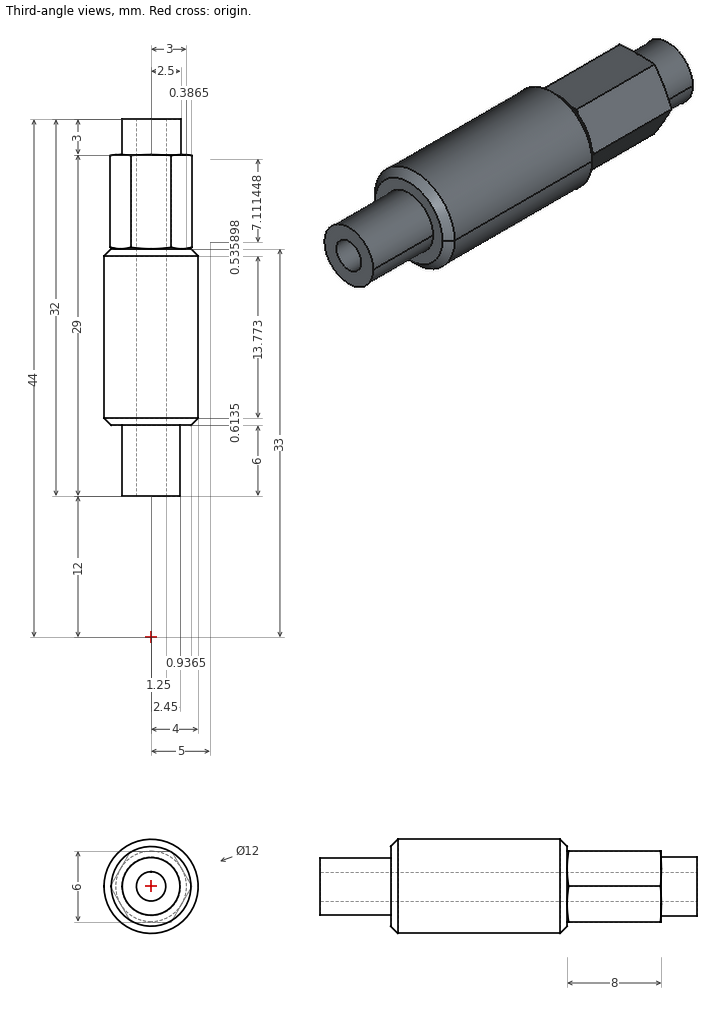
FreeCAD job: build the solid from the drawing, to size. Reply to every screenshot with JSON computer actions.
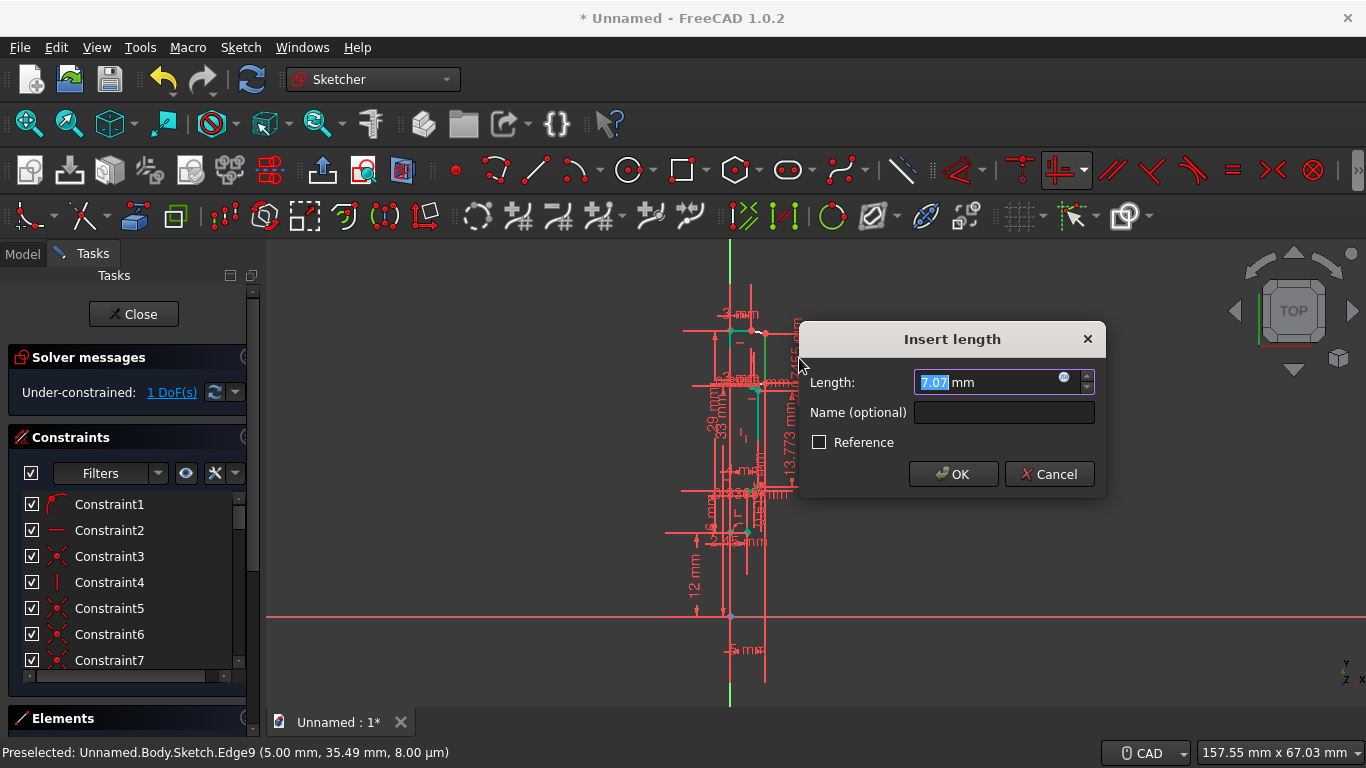
{"action": "type", "text": "7.111448"}
{"action": "key", "text": "Return"}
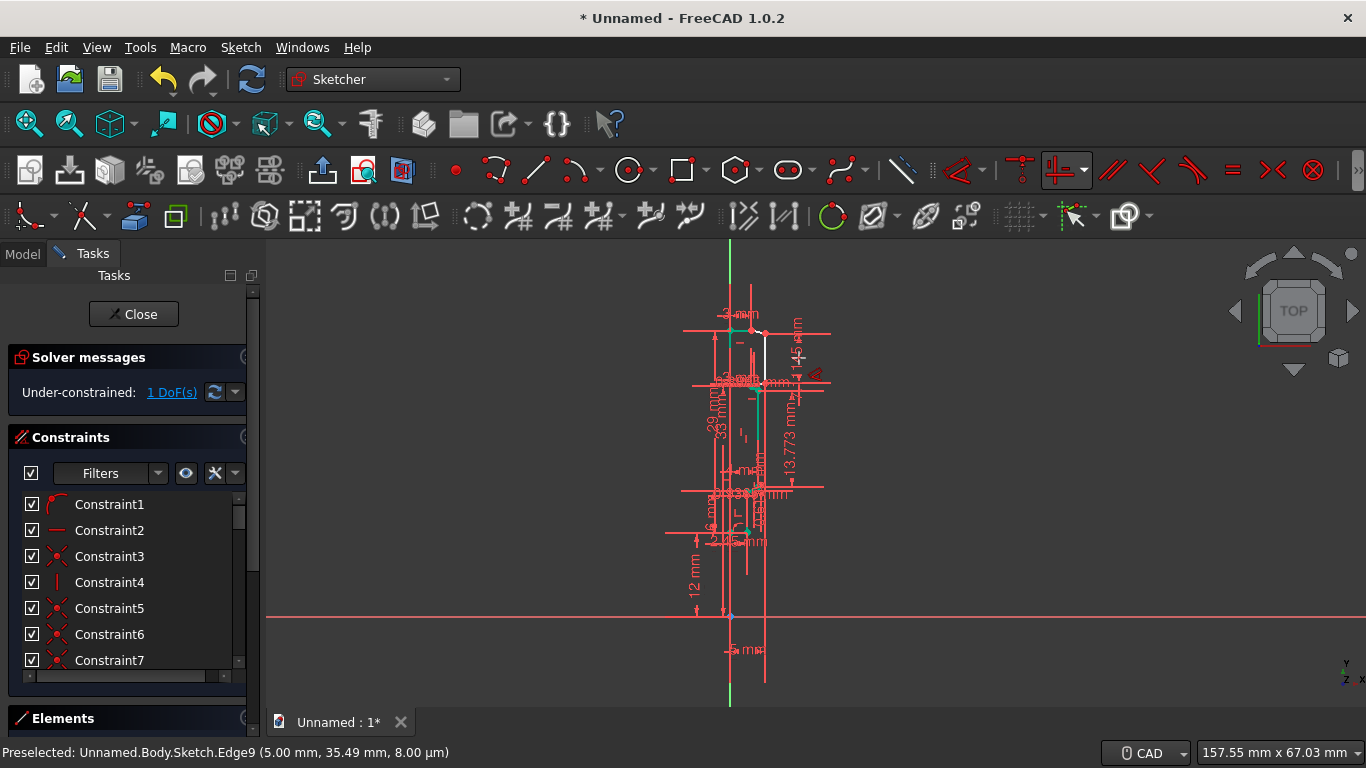
{"action": "scroll", "coordinate": [760, 384], "scroll_direction": "up", "scroll_amount": 12}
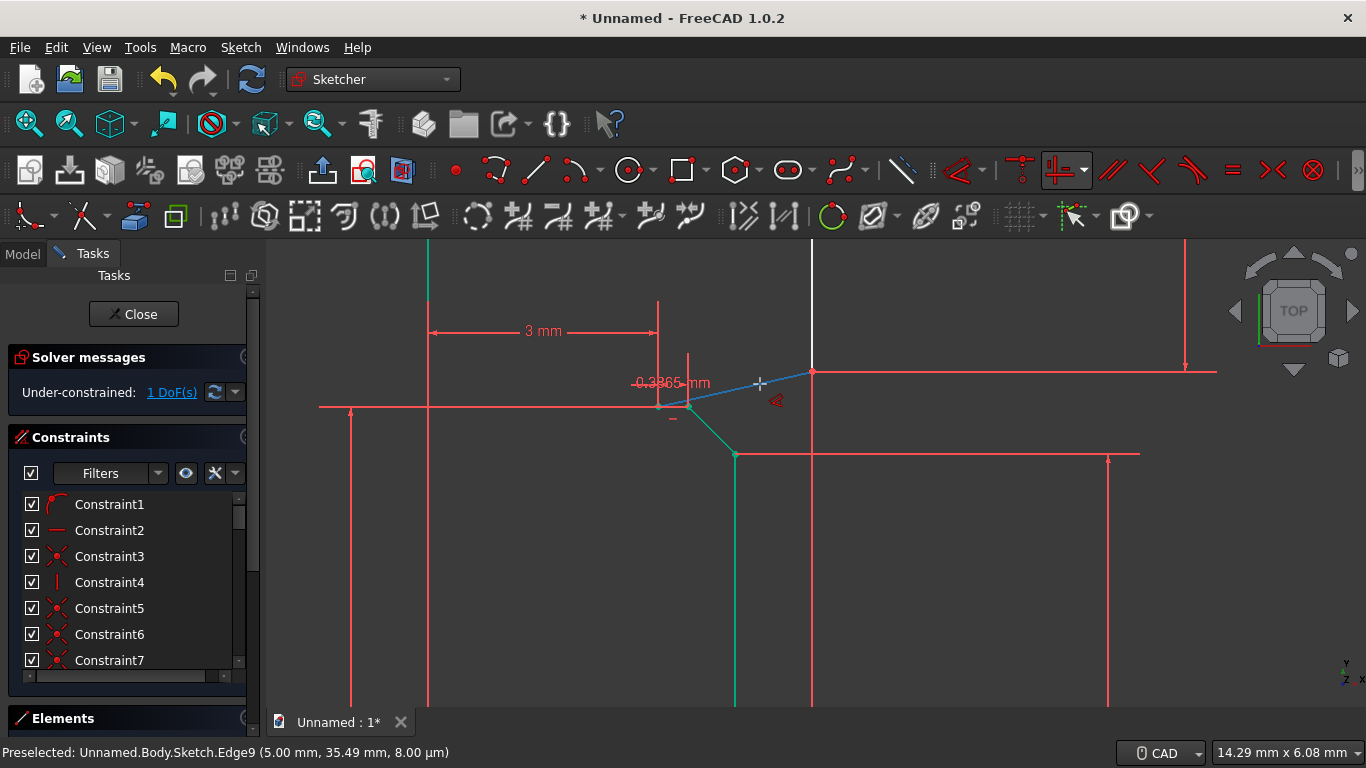
{"action": "left_click", "coordinate": [751, 386]}
{"action": "left_click", "coordinate": [846, 389]}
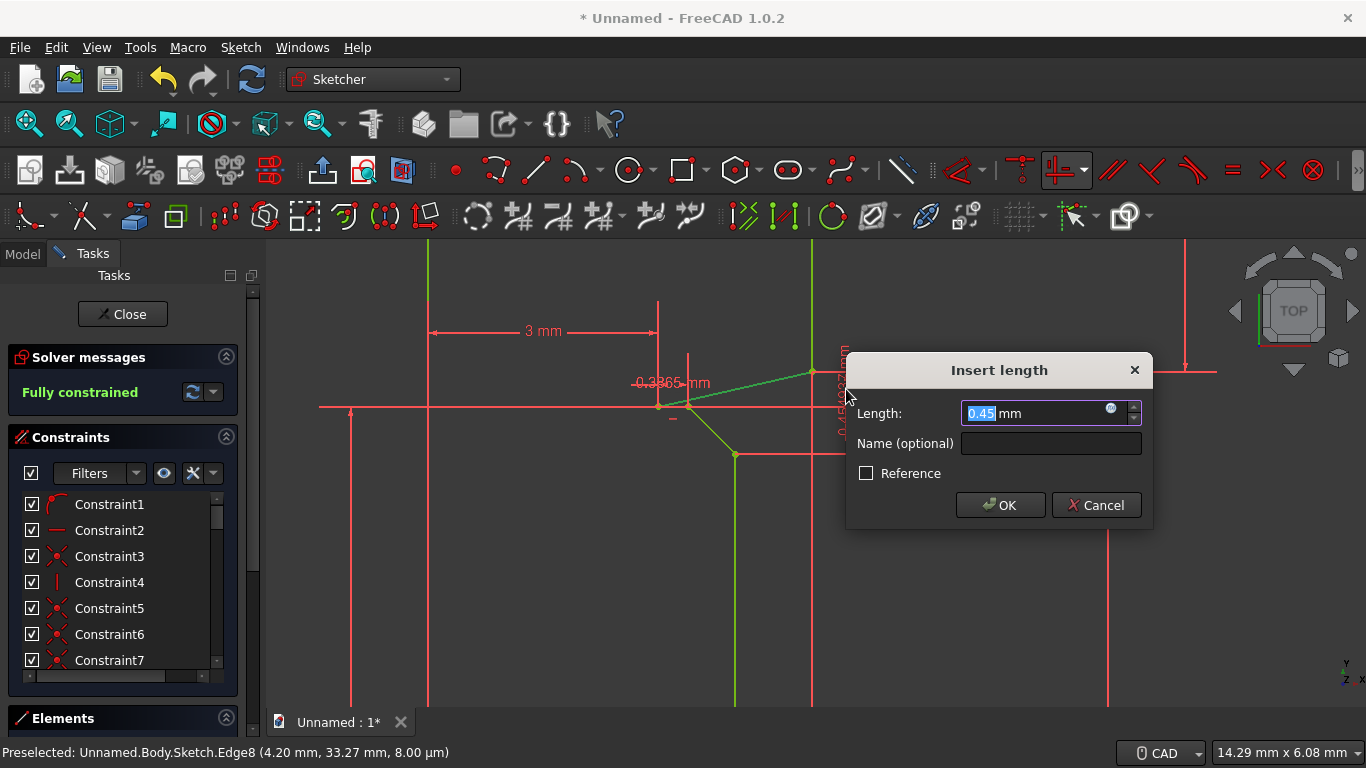
{"action": "type", "text": "0.535898"}
{"action": "key", "text": "Return"}
{"action": "key", "text": "Escape"}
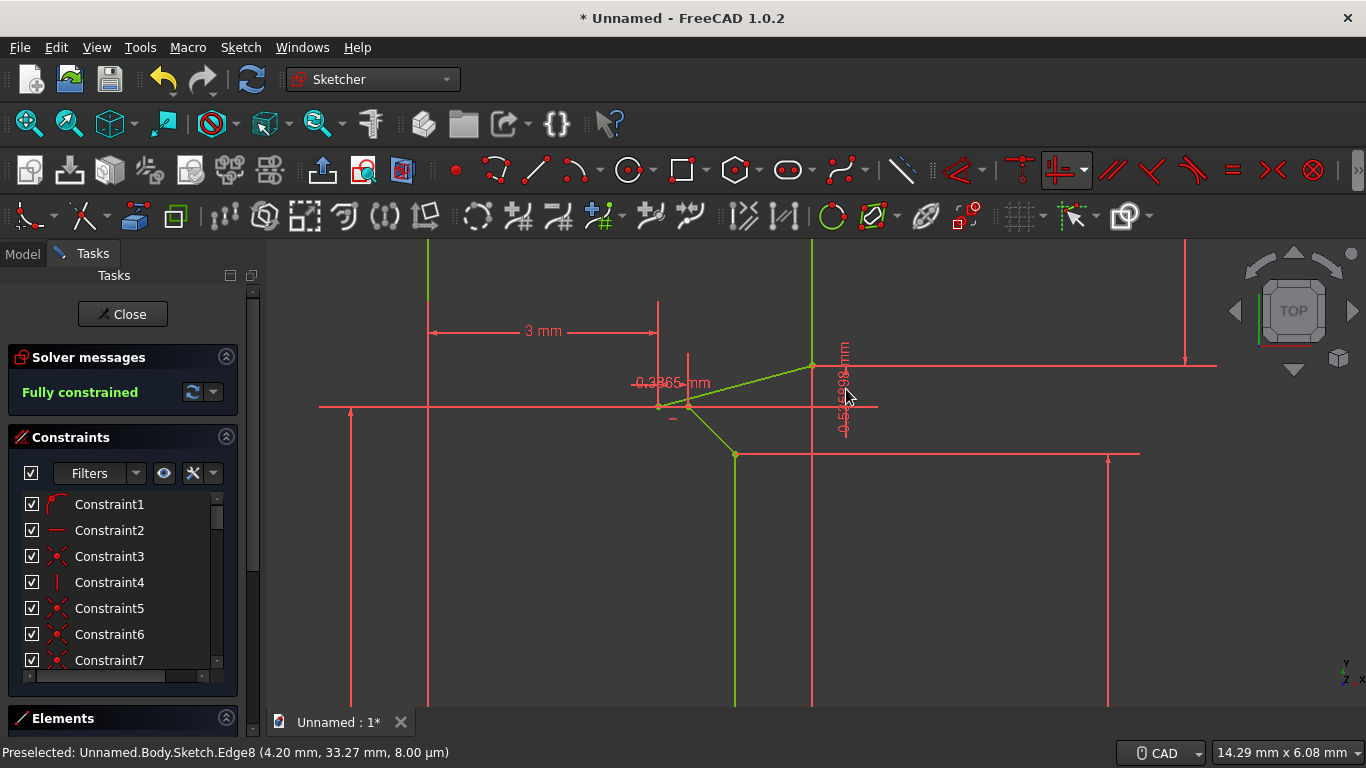
{"action": "left_click", "coordinate": [123, 314]}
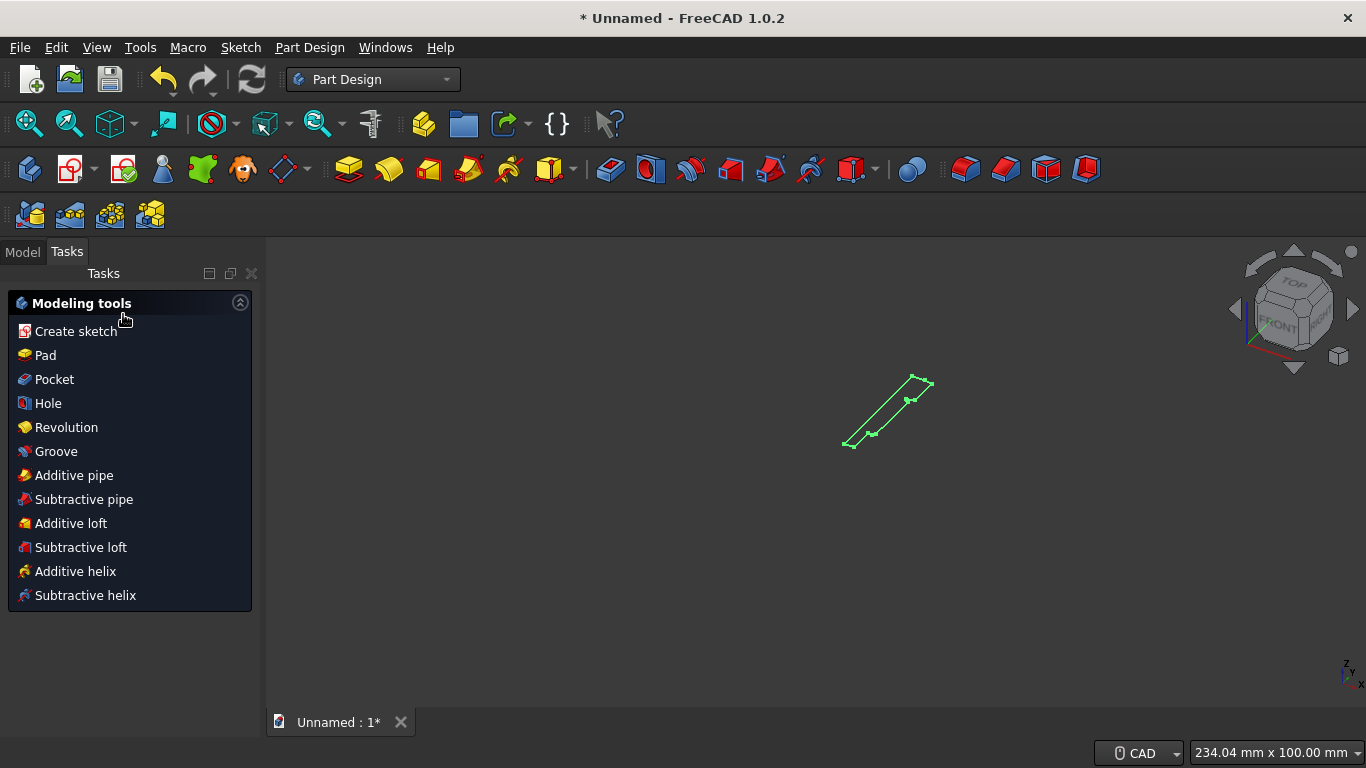
{"action": "left_click", "coordinate": [390, 170]}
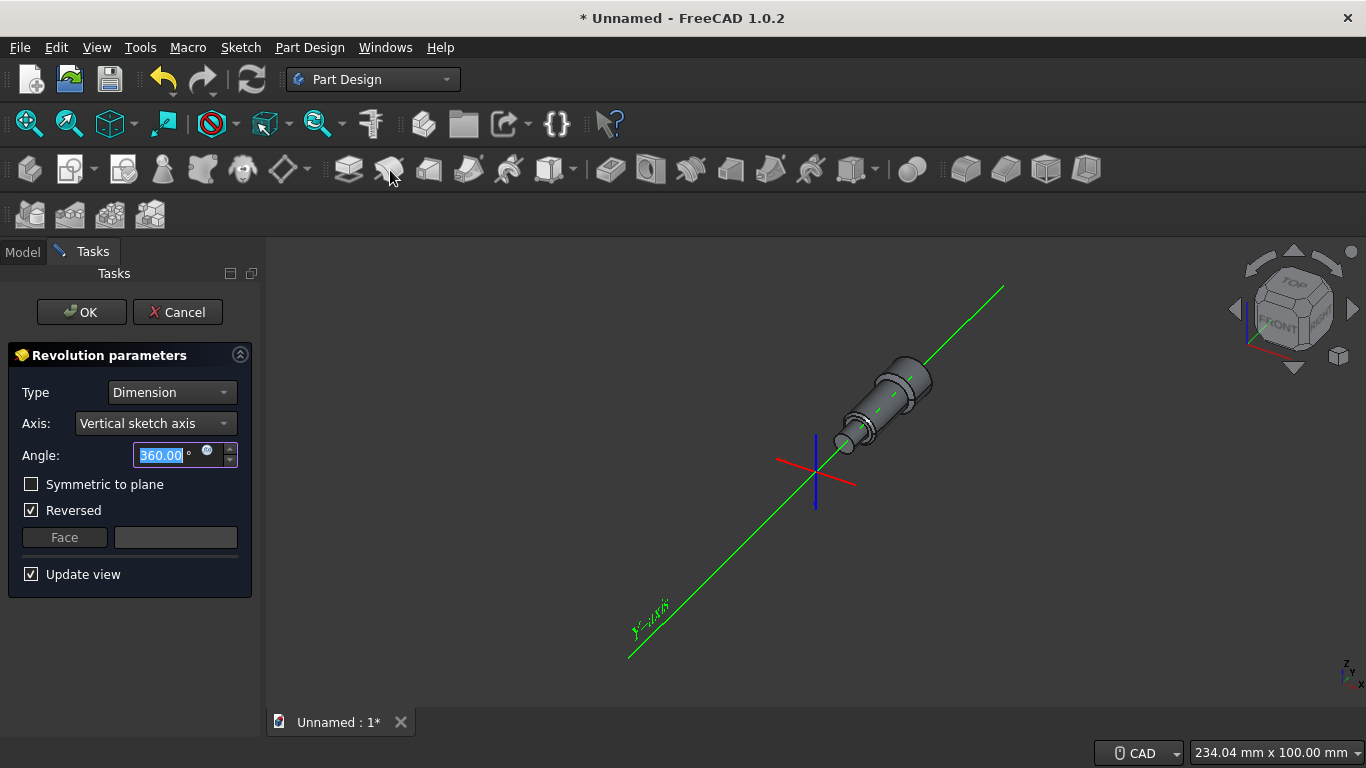
{"action": "left_click", "coordinate": [82, 312]}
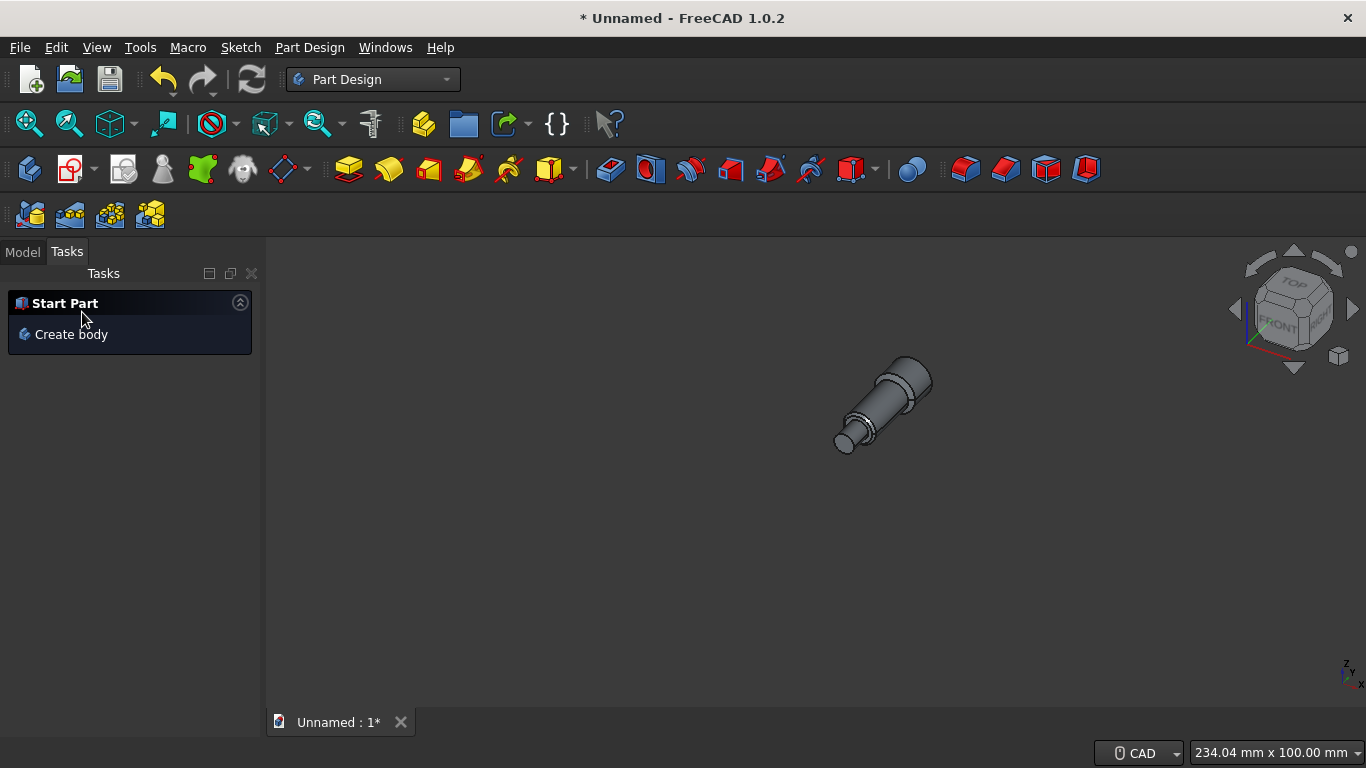
{"action": "left_click", "coordinate": [30, 124]}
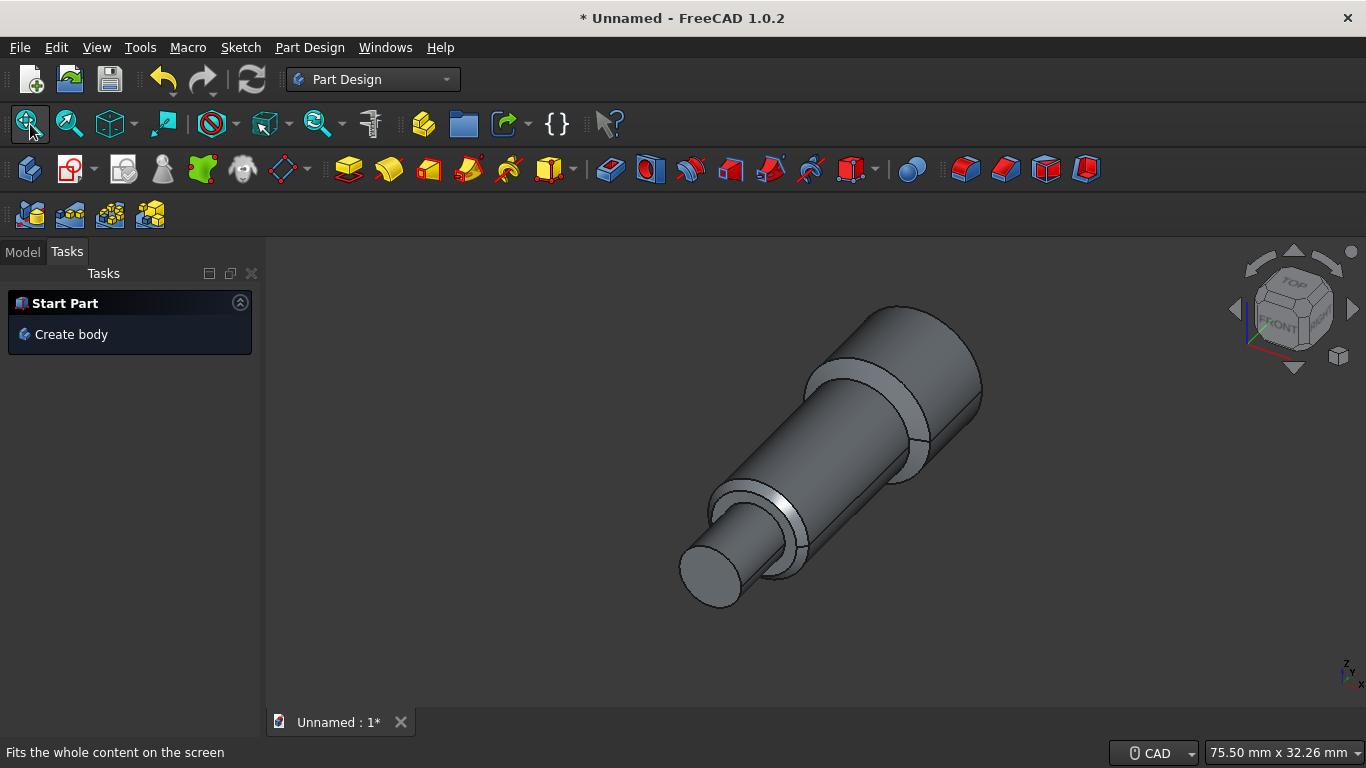
{"action": "left_click", "coordinate": [23, 251]}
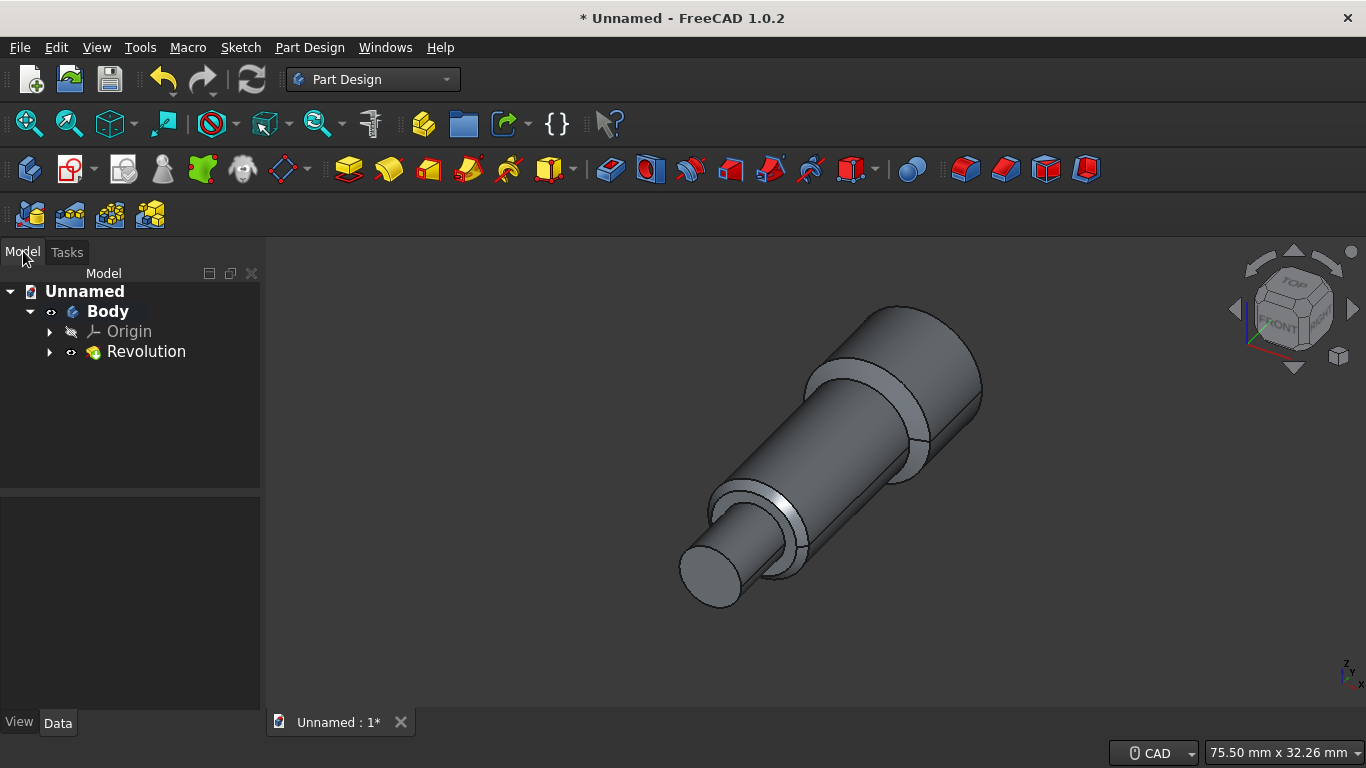
{"action": "left_click", "coordinate": [50, 332]}